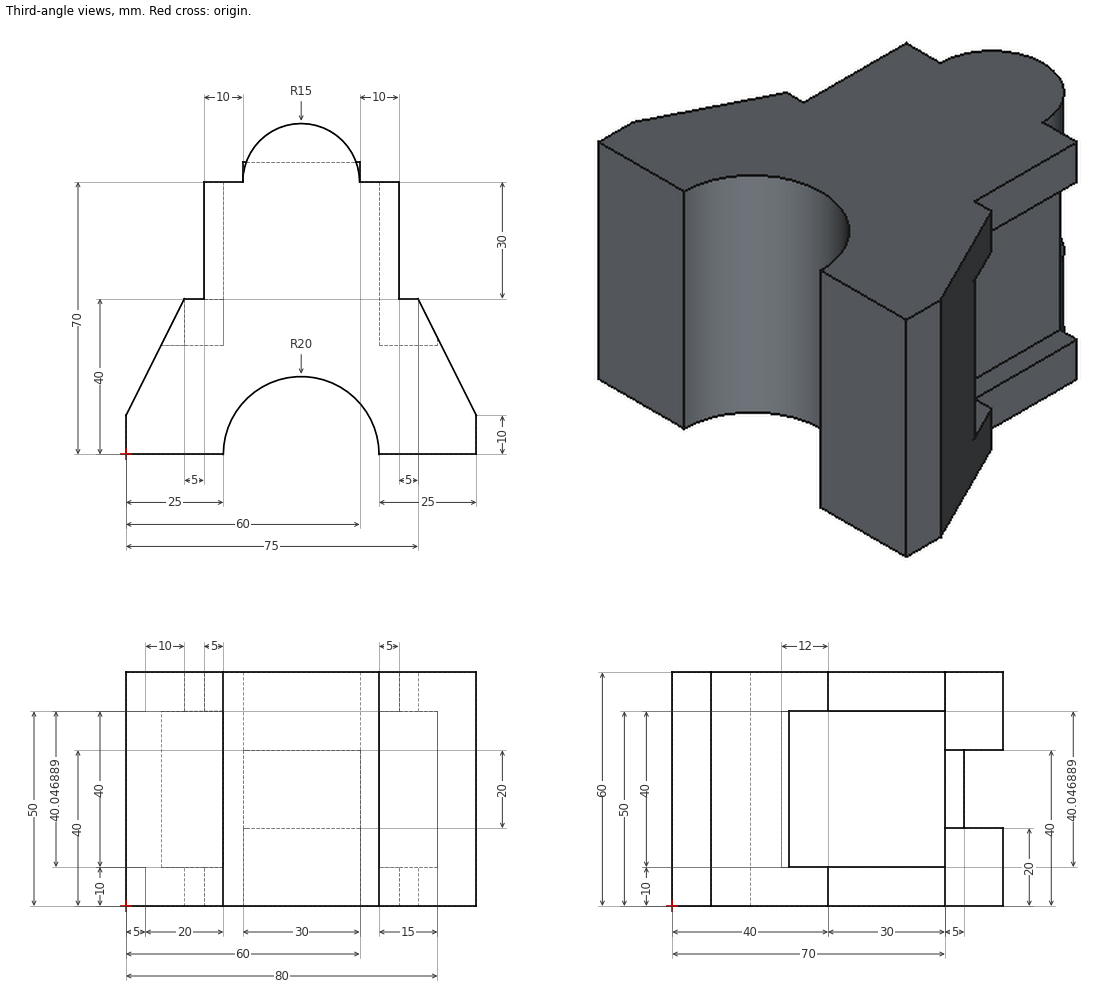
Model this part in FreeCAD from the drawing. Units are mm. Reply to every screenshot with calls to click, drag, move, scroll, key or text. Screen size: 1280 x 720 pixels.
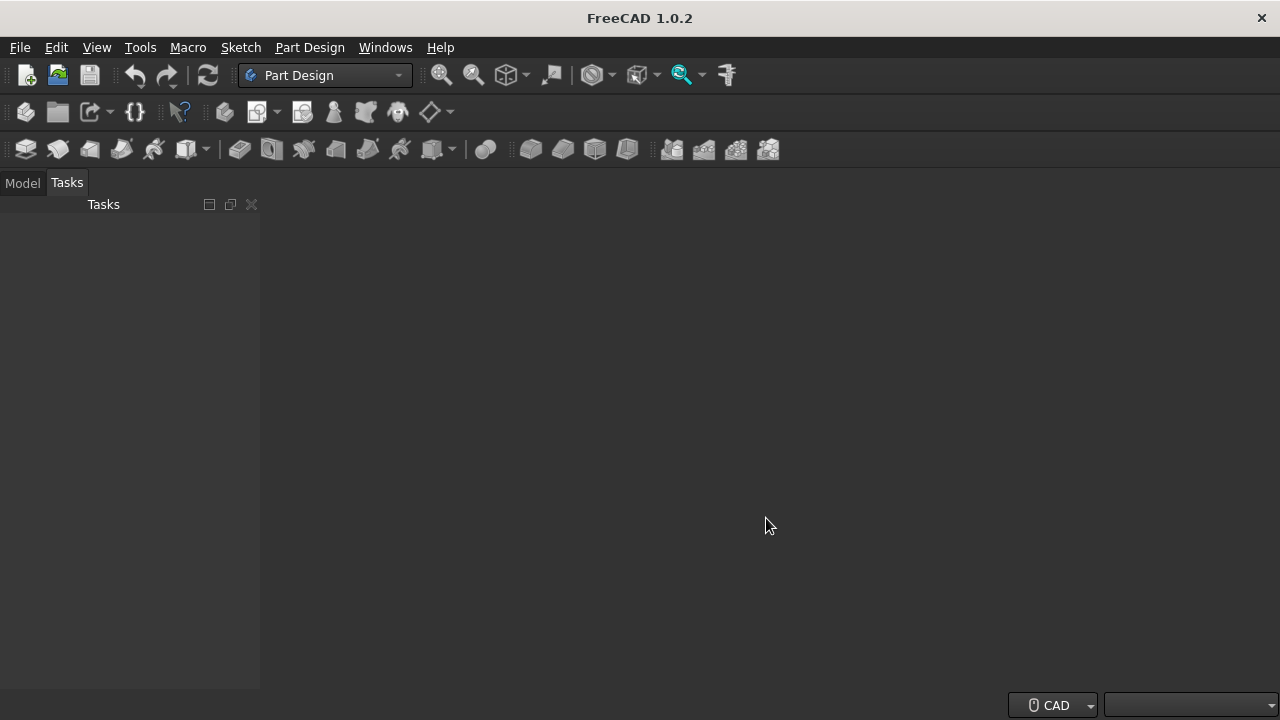
click(26, 76)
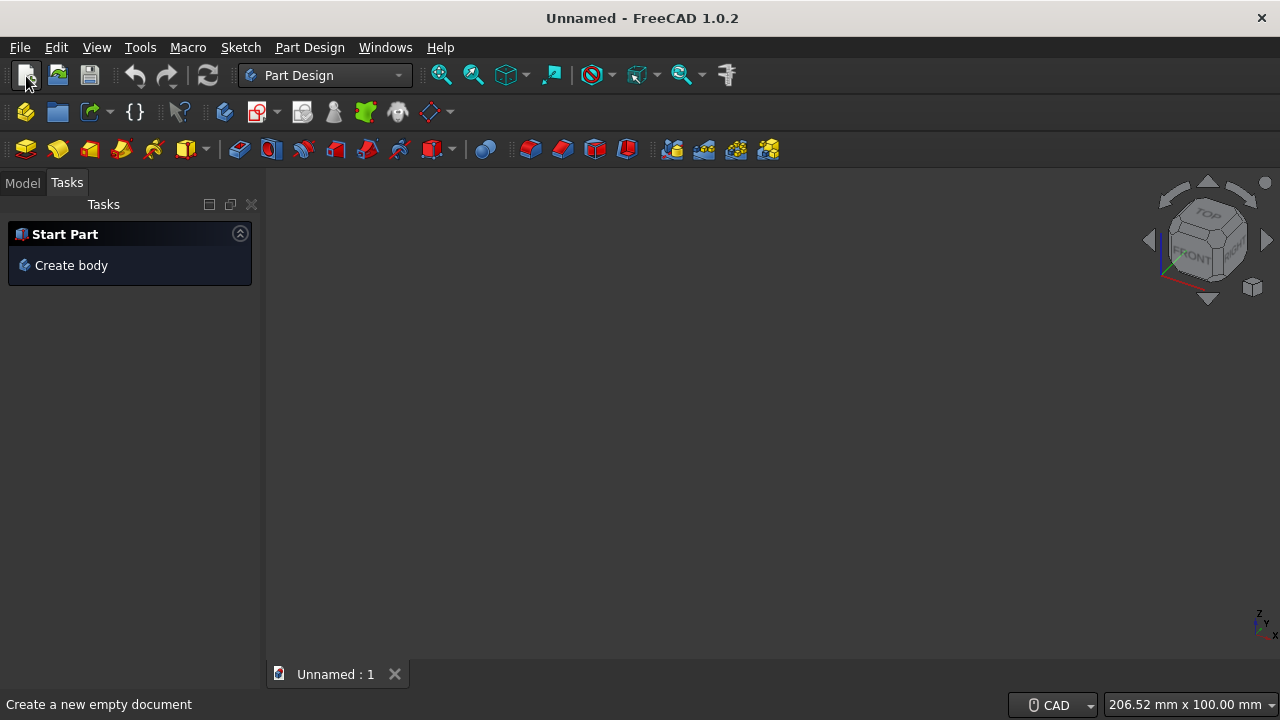
click(258, 112)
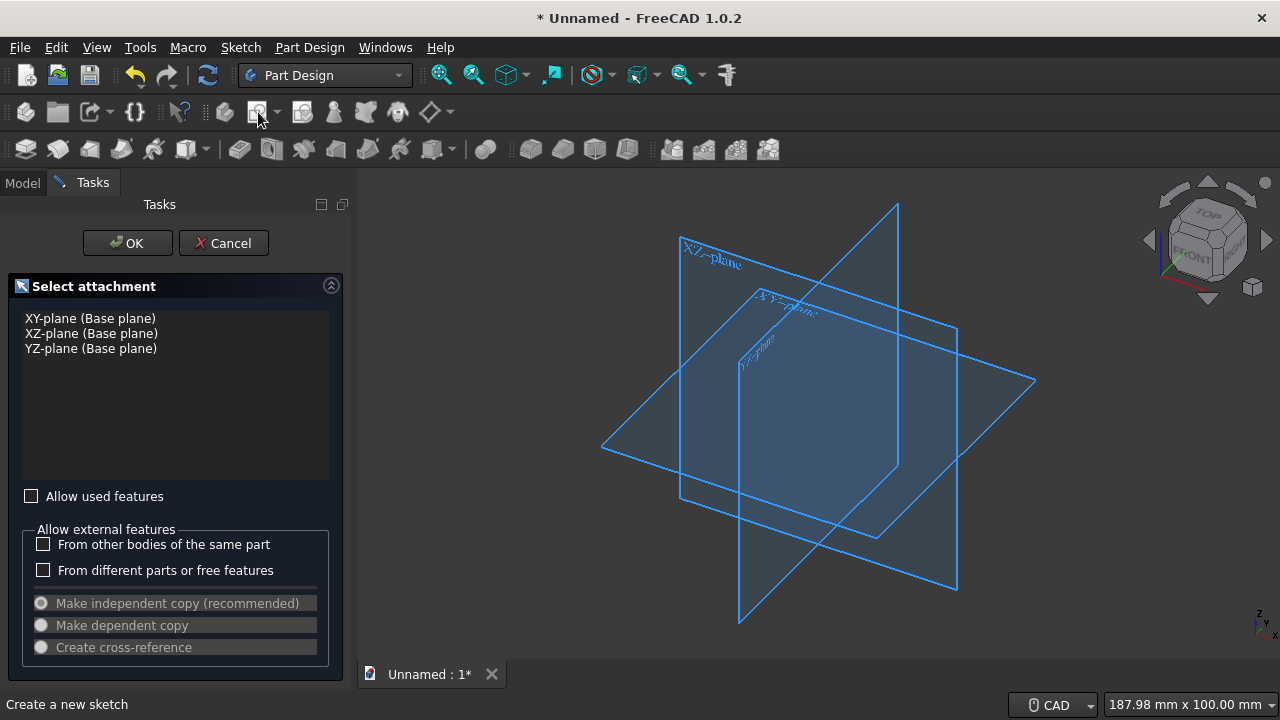
click(82, 318)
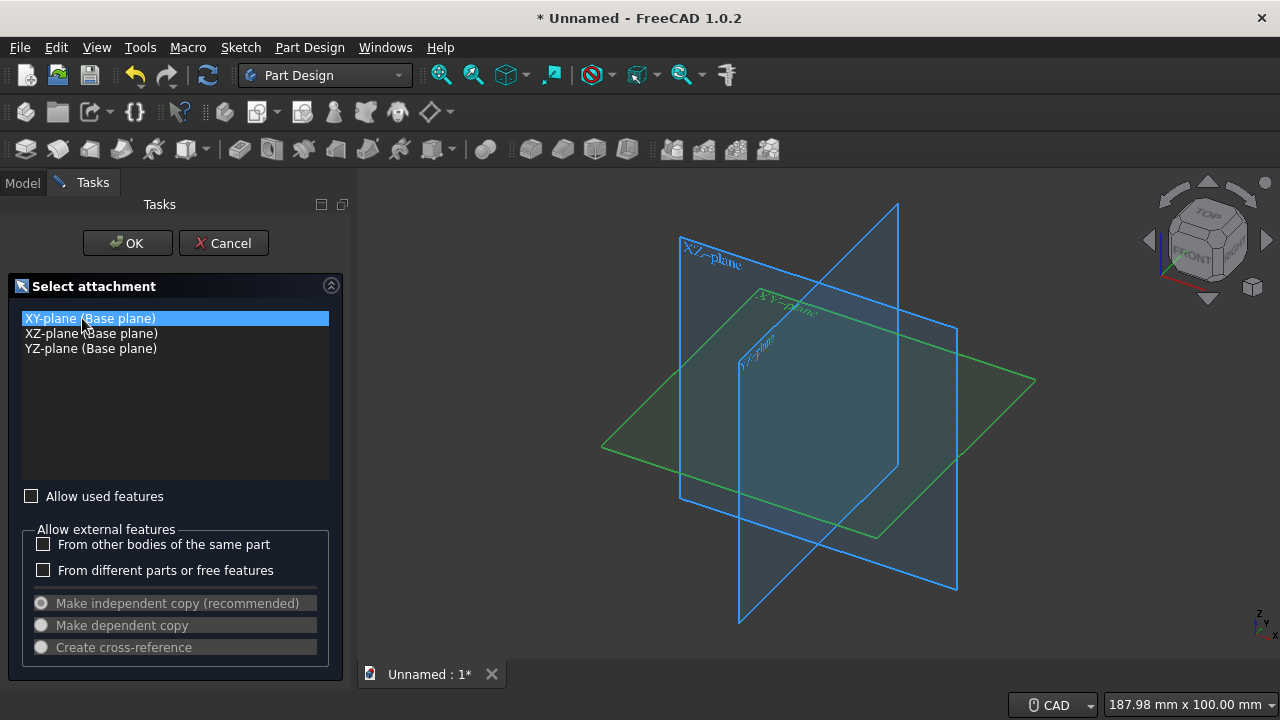
click(128, 243)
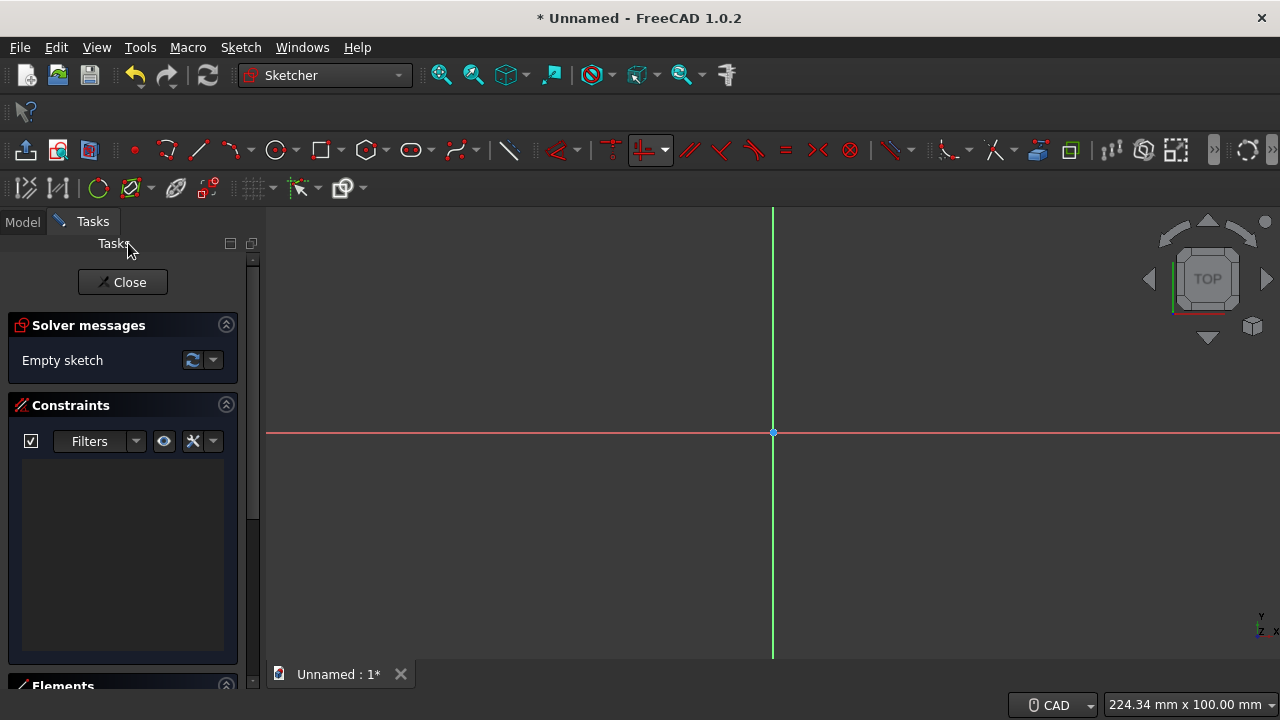
scroll(374, 631, down, 3)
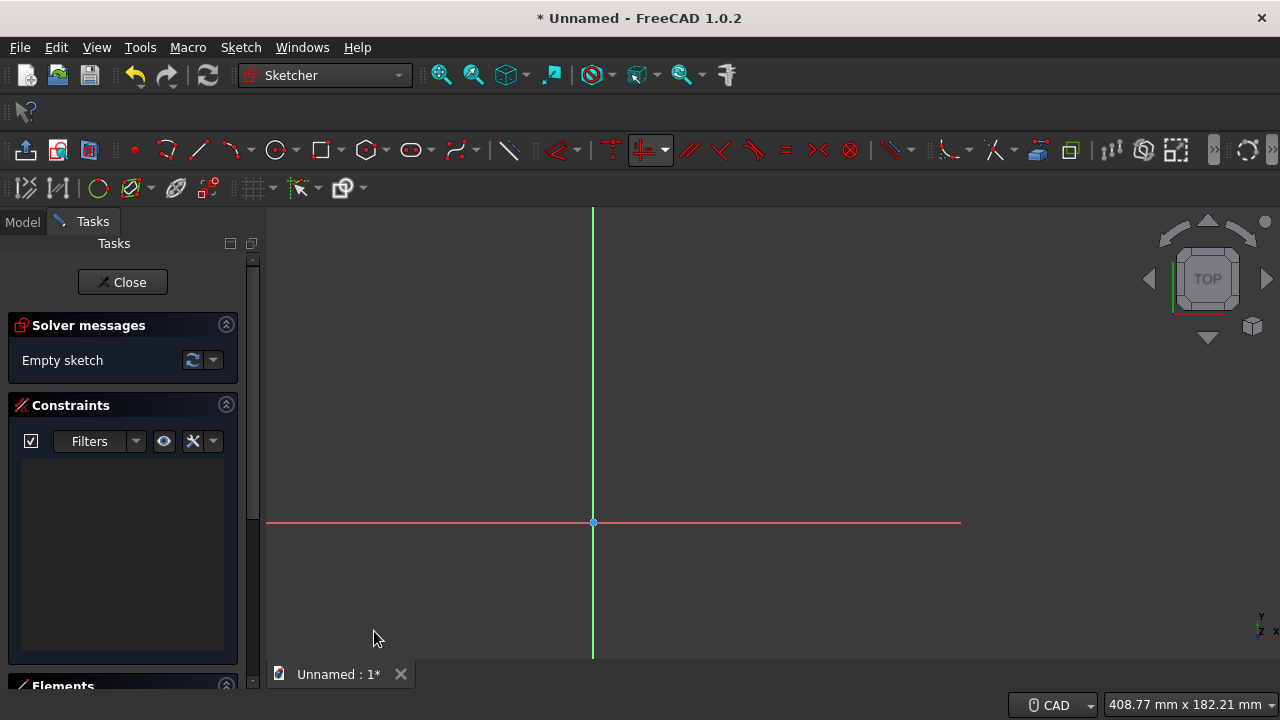
key(g)
key(m)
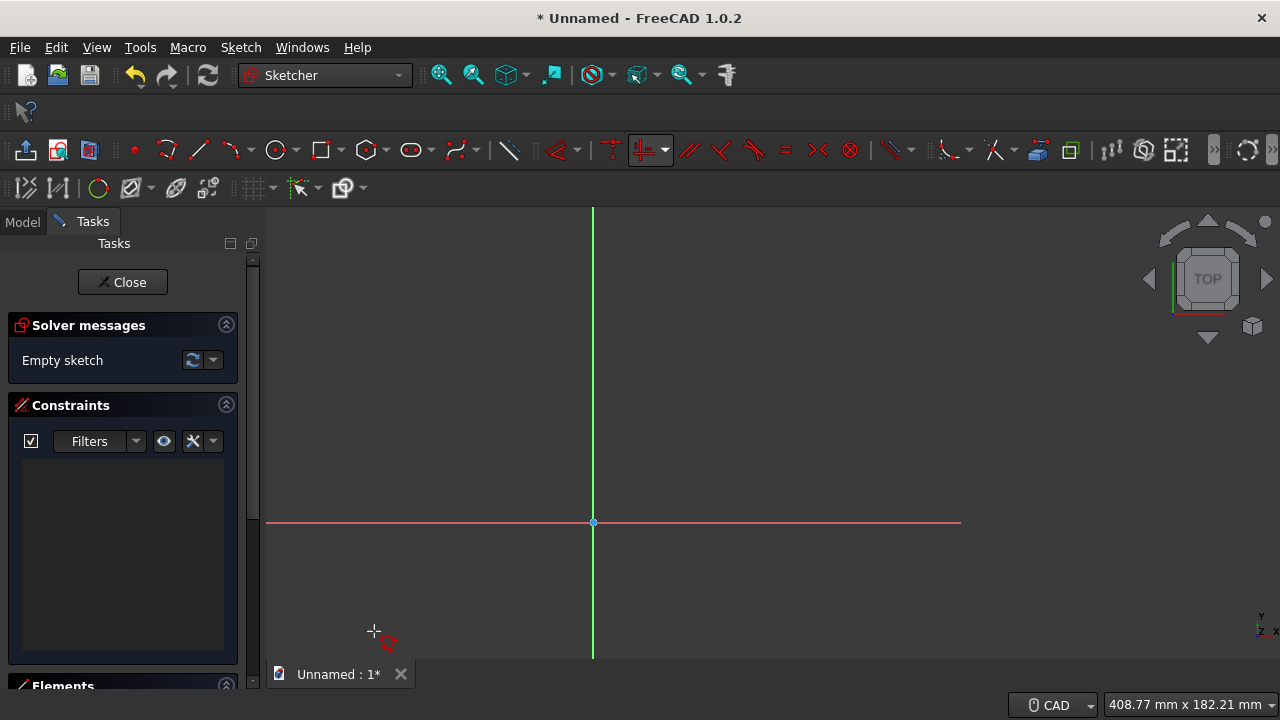
click(754, 523)
click(816, 514)
click(816, 498)
click(779, 424)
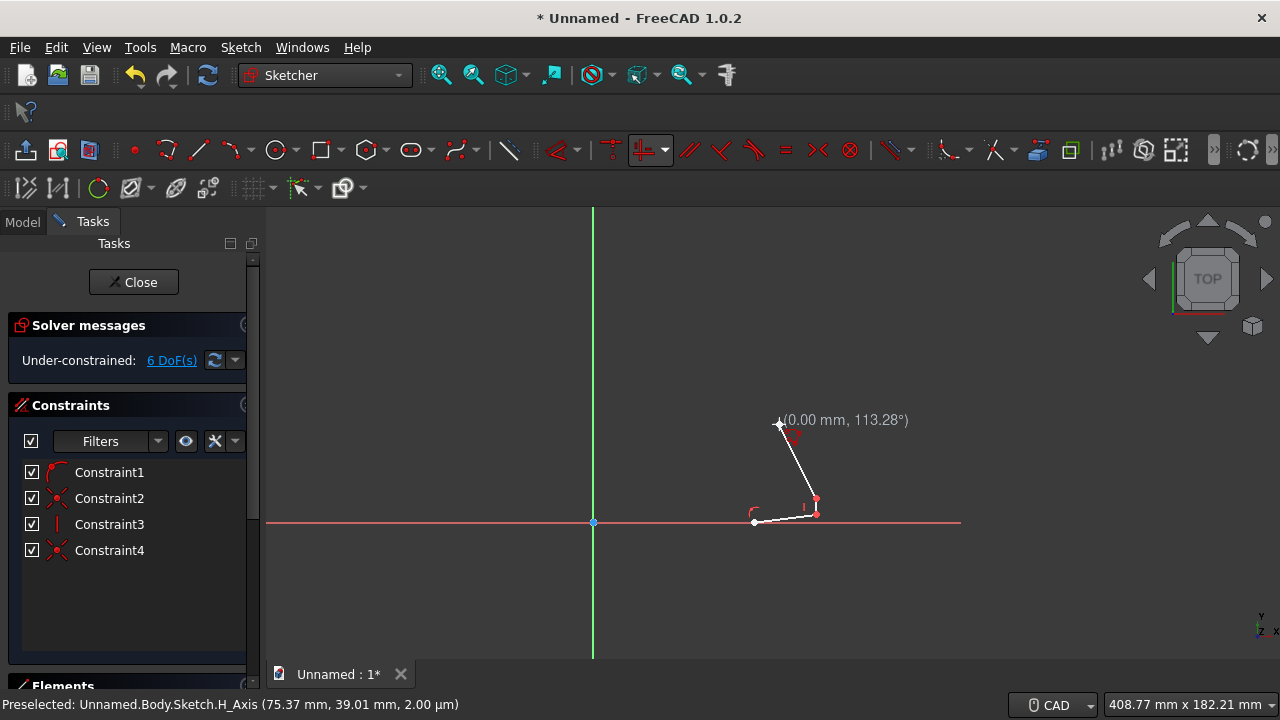
scroll(767, 424, up, 2)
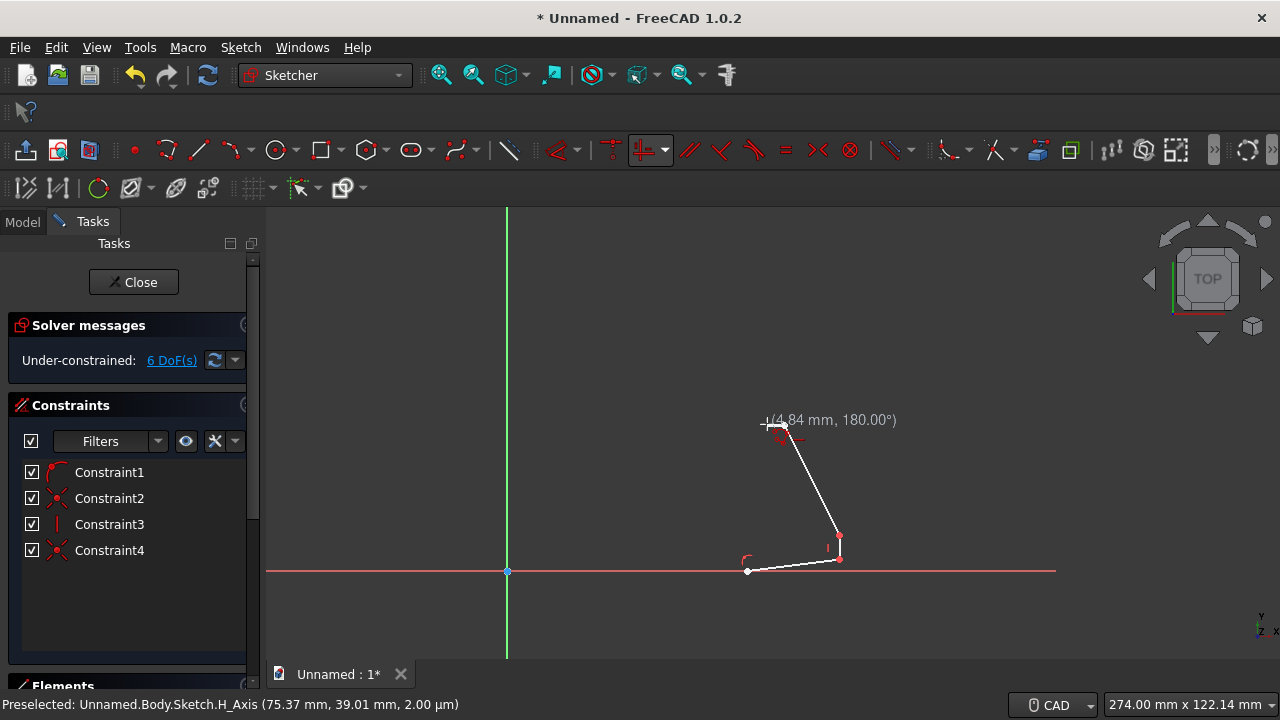
click(766, 424)
click(766, 312)
click(729, 312)
right_click(729, 312)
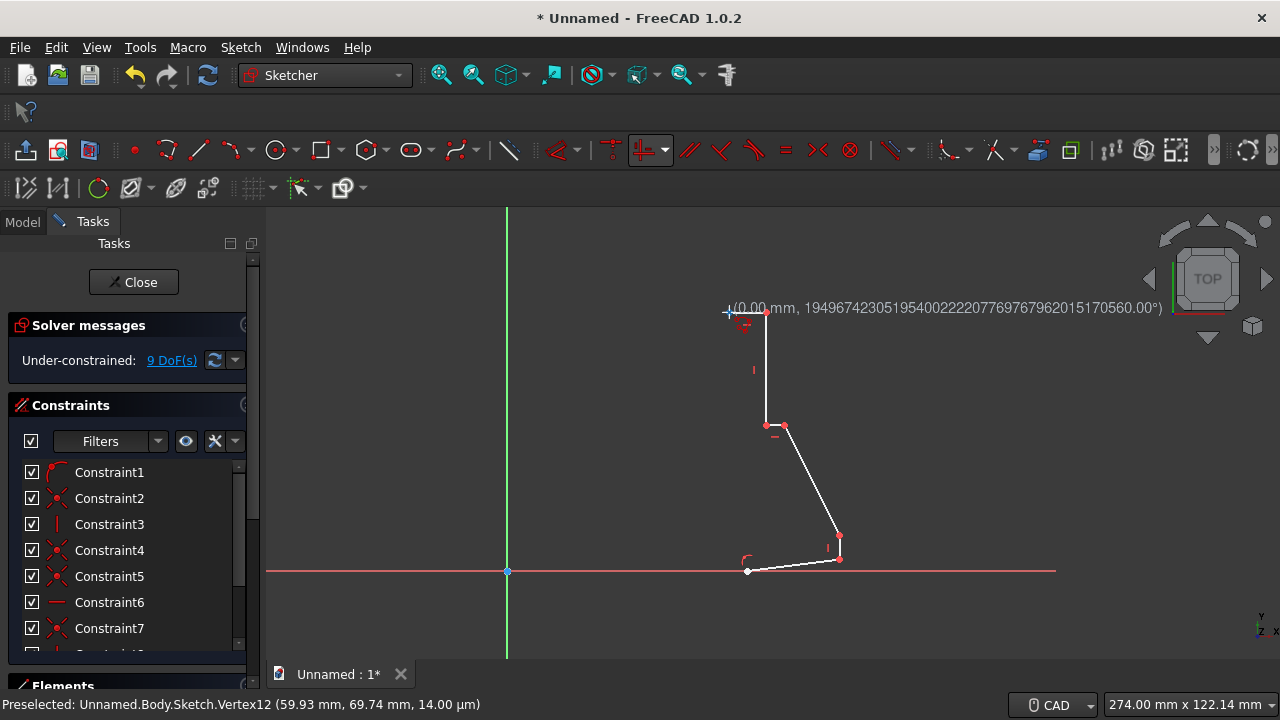
click(618, 312)
click(581, 312)
click(581, 423)
click(563, 423)
click(507, 534)
click(507, 571)
click(600, 562)
right_click(600, 562)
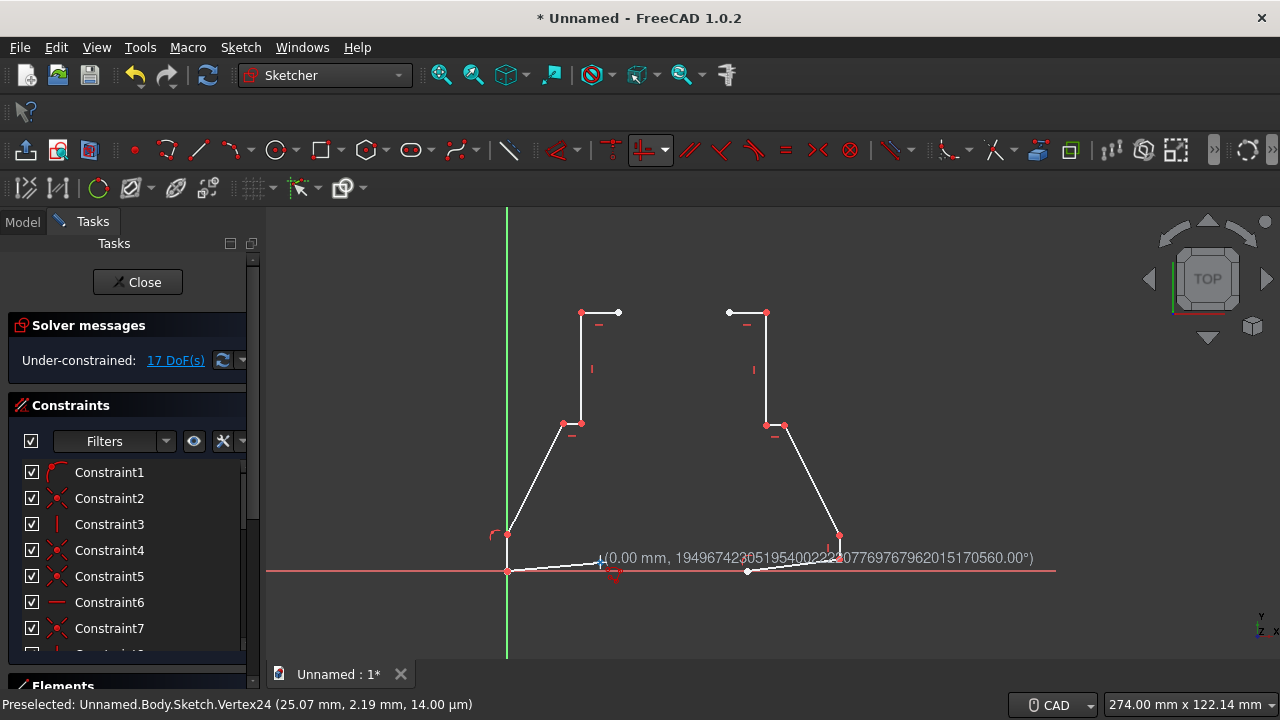
key(g)
key(3)
key(a)